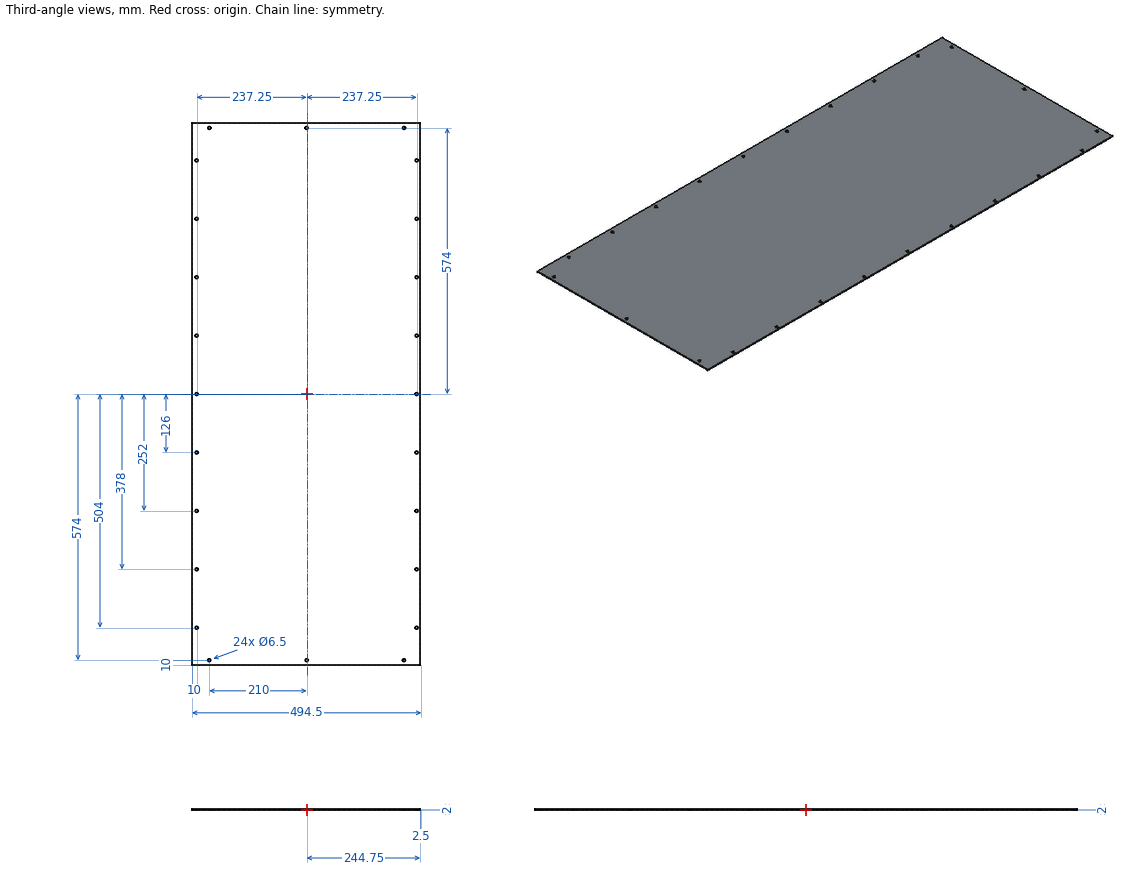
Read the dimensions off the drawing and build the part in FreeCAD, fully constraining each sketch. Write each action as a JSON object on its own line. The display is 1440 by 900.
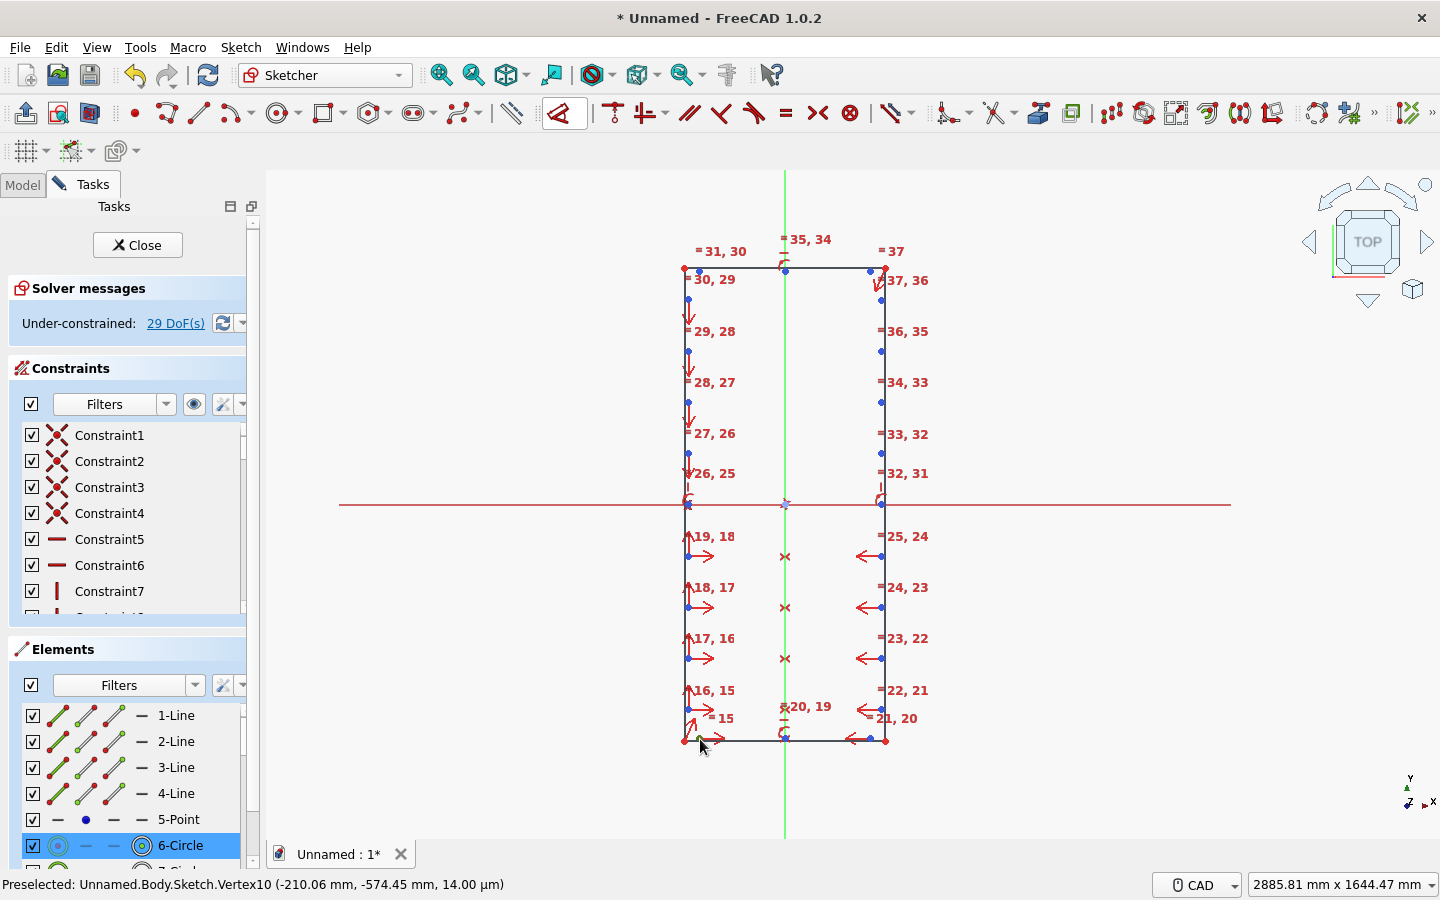
{"action": "left_click", "coordinate": [700, 272]}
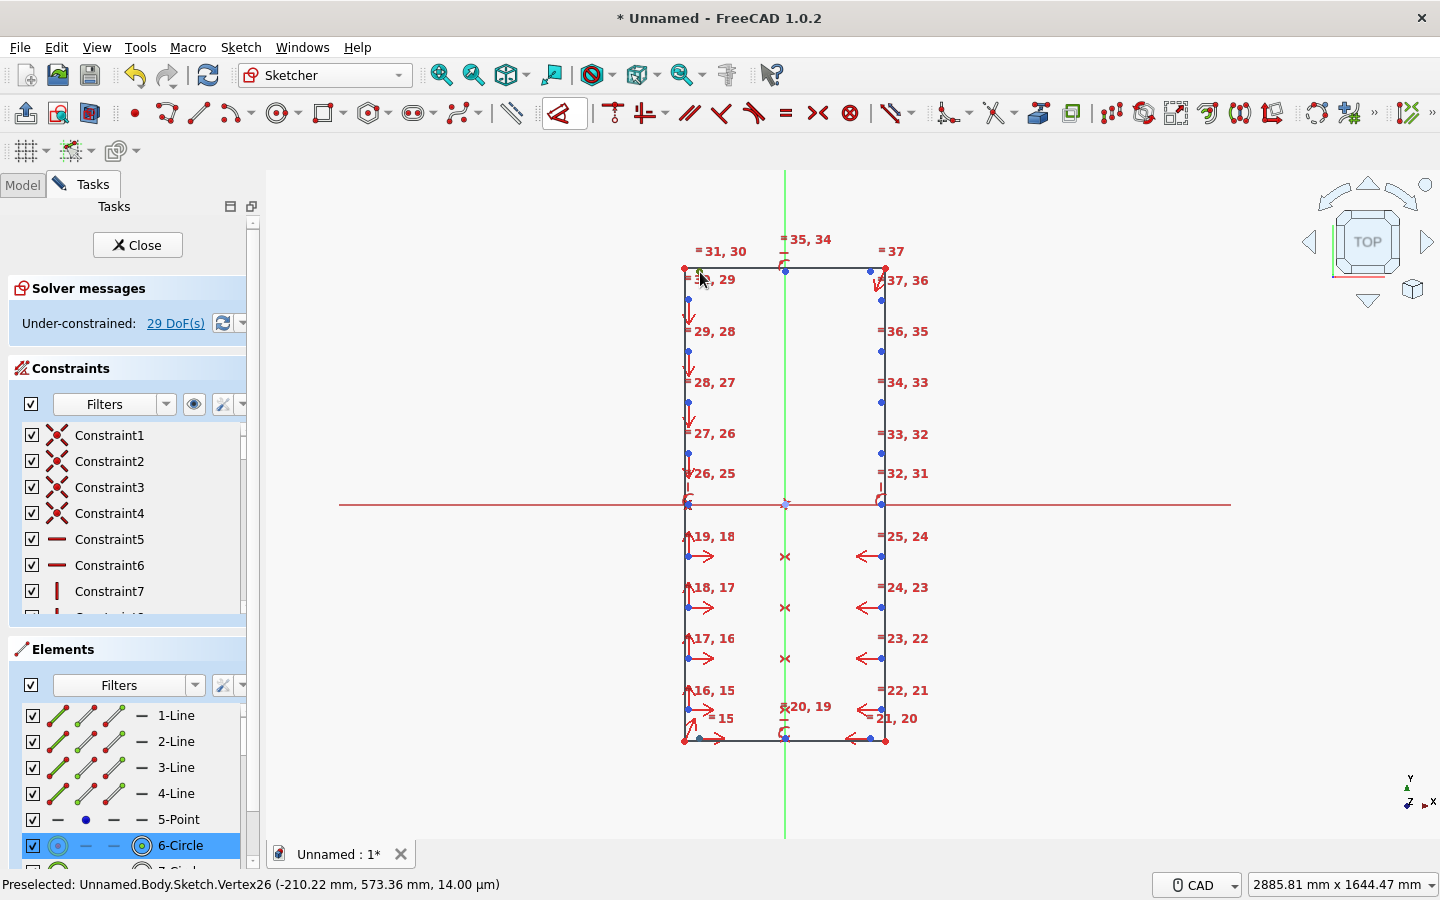
{"action": "left_click", "coordinate": [364, 505]}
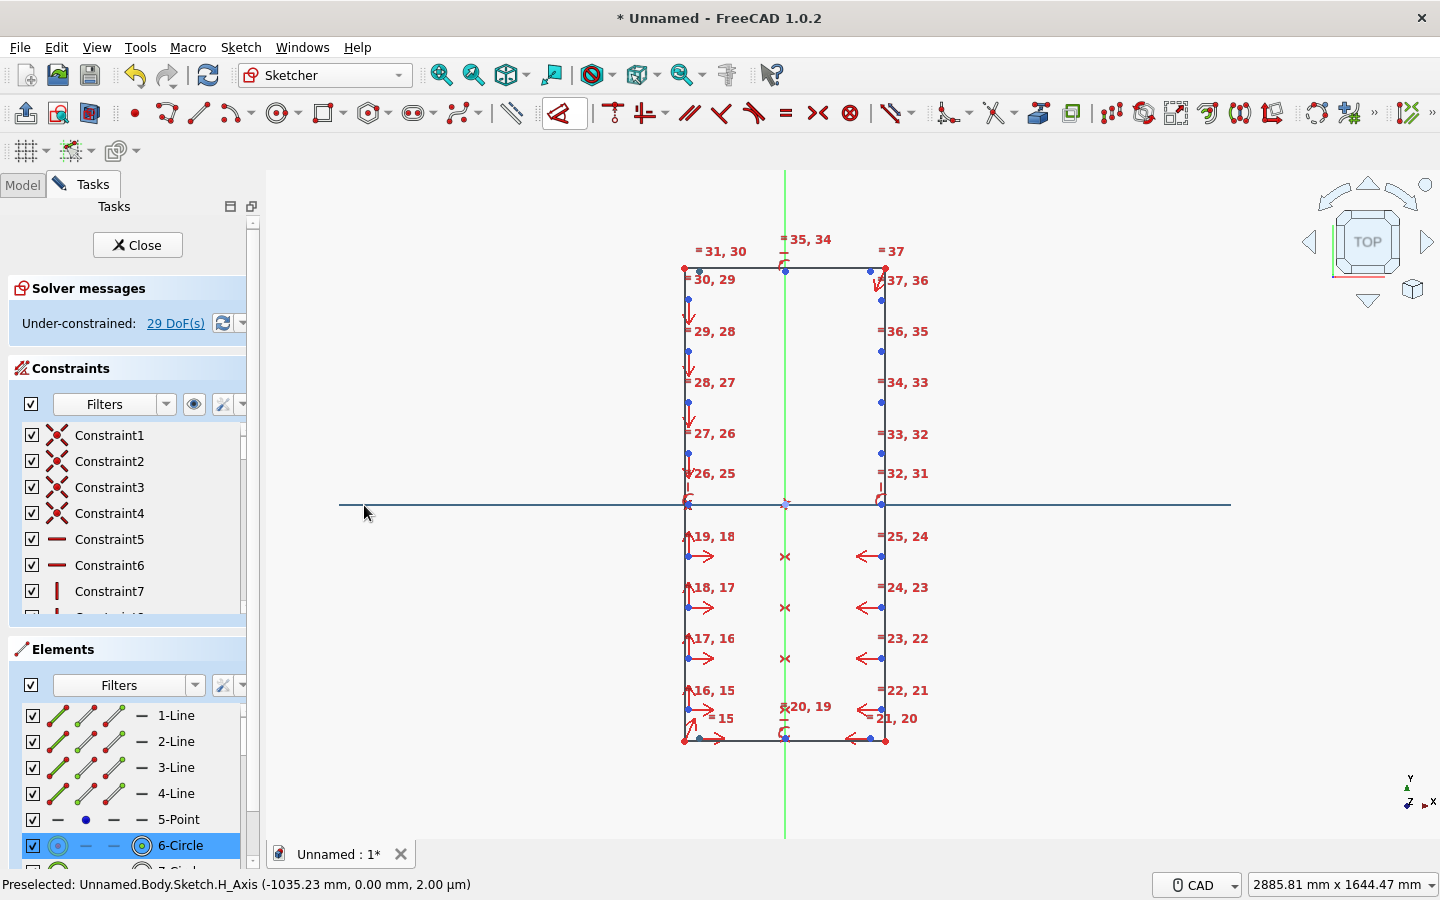
{"action": "key", "text": "s"}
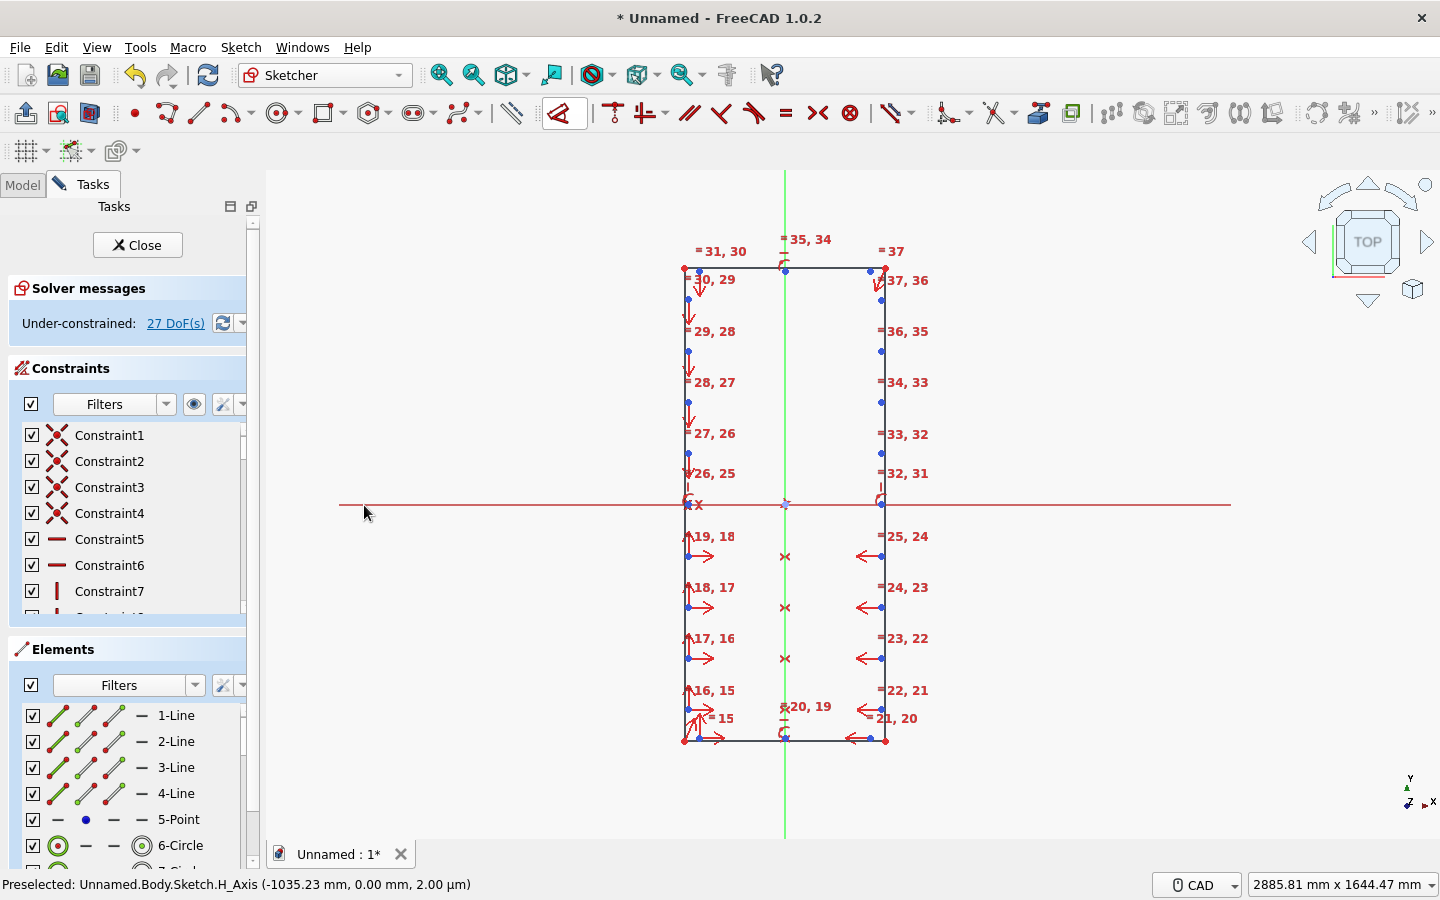
{"action": "left_click", "coordinate": [882, 556]}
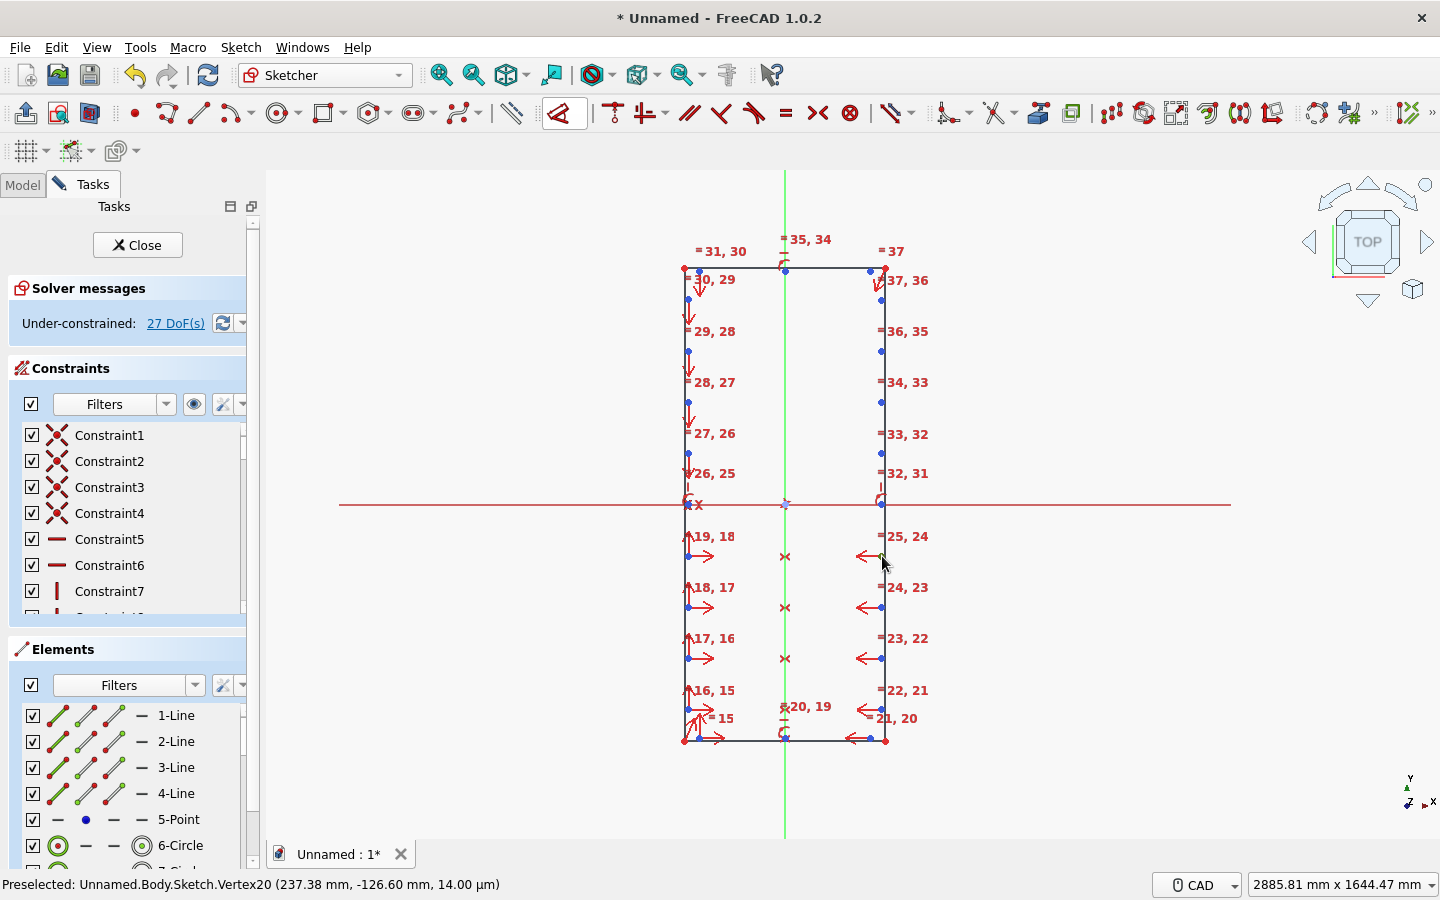
{"action": "left_click", "coordinate": [882, 454]}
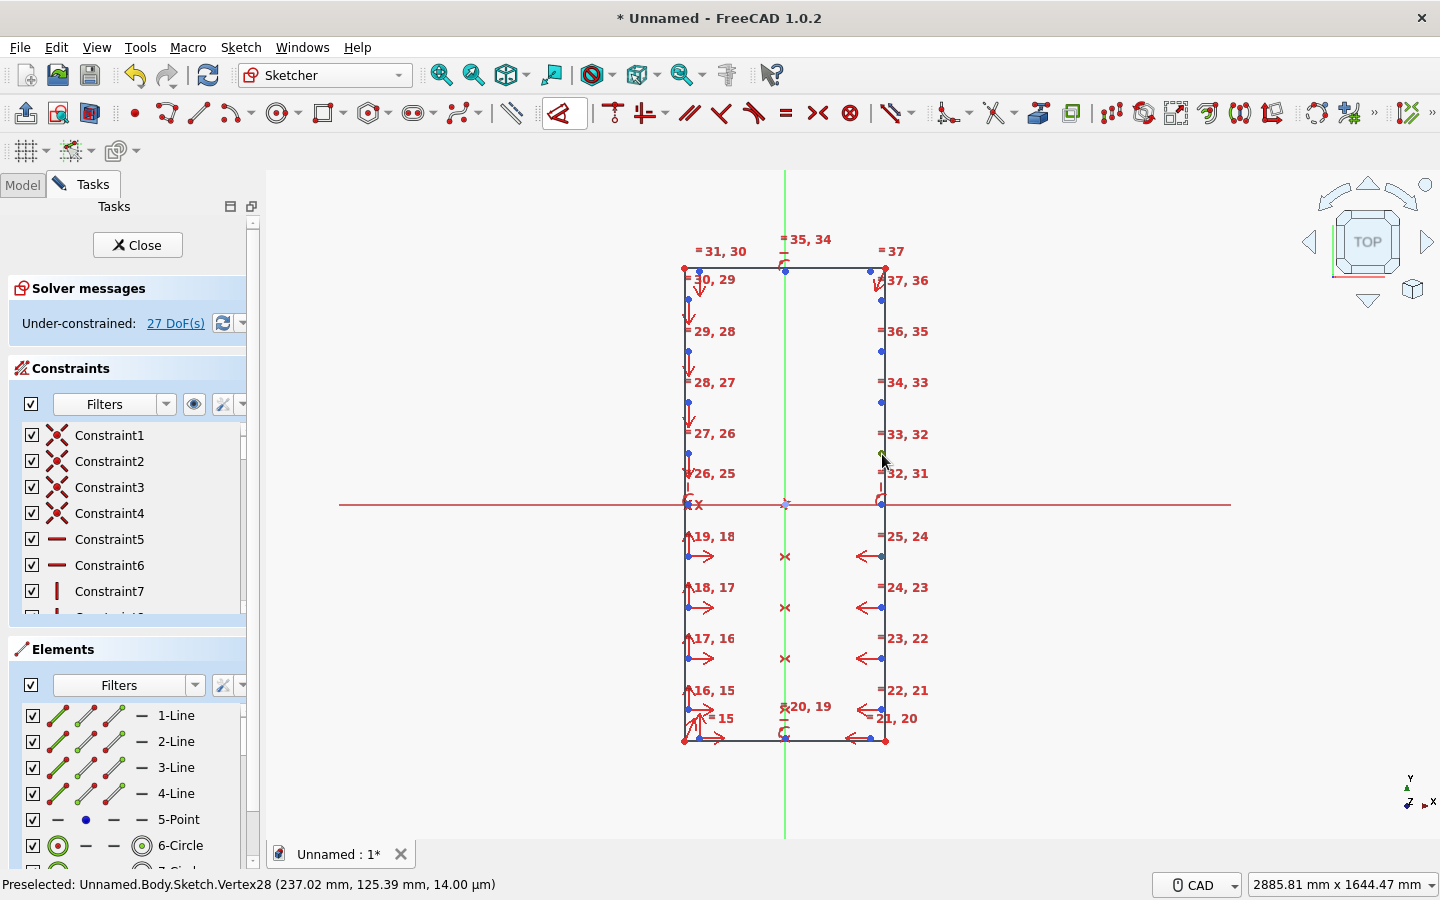
{"action": "left_click", "coordinate": [364, 505]}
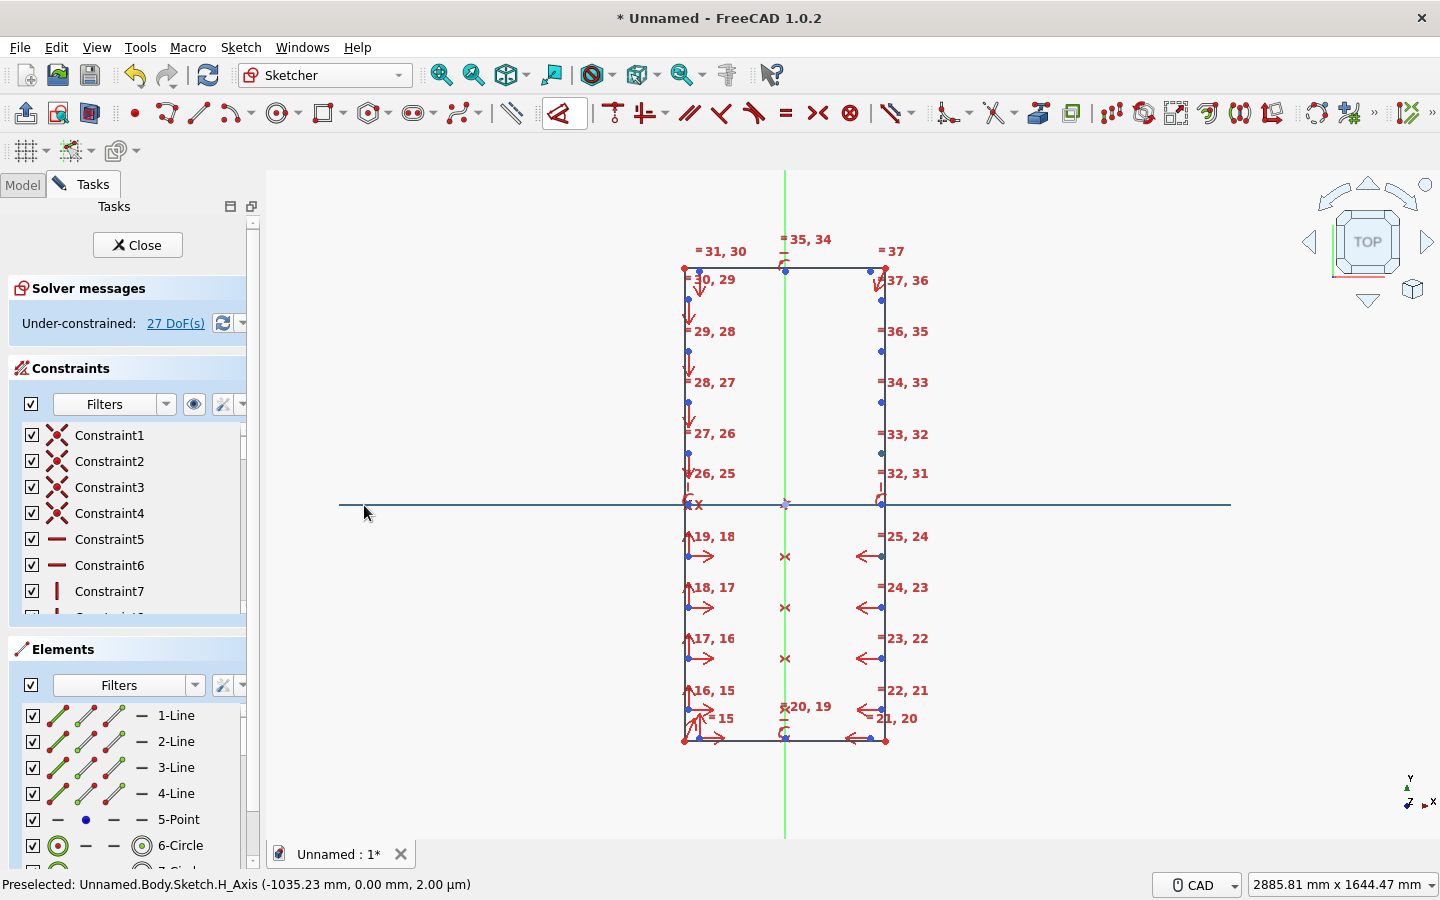
{"action": "key", "text": "s"}